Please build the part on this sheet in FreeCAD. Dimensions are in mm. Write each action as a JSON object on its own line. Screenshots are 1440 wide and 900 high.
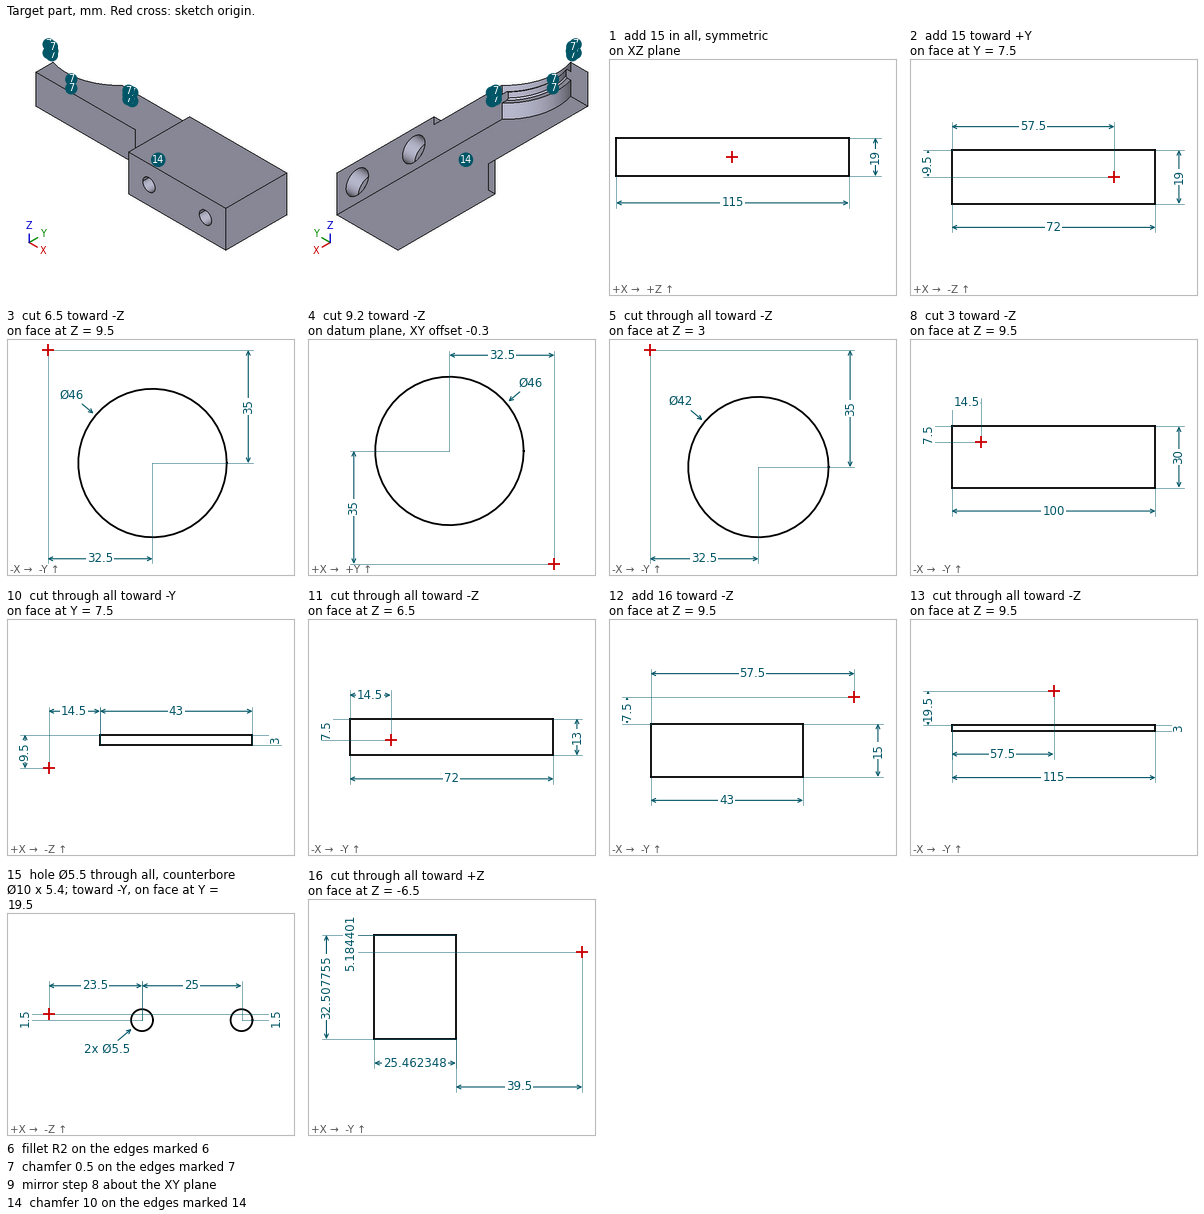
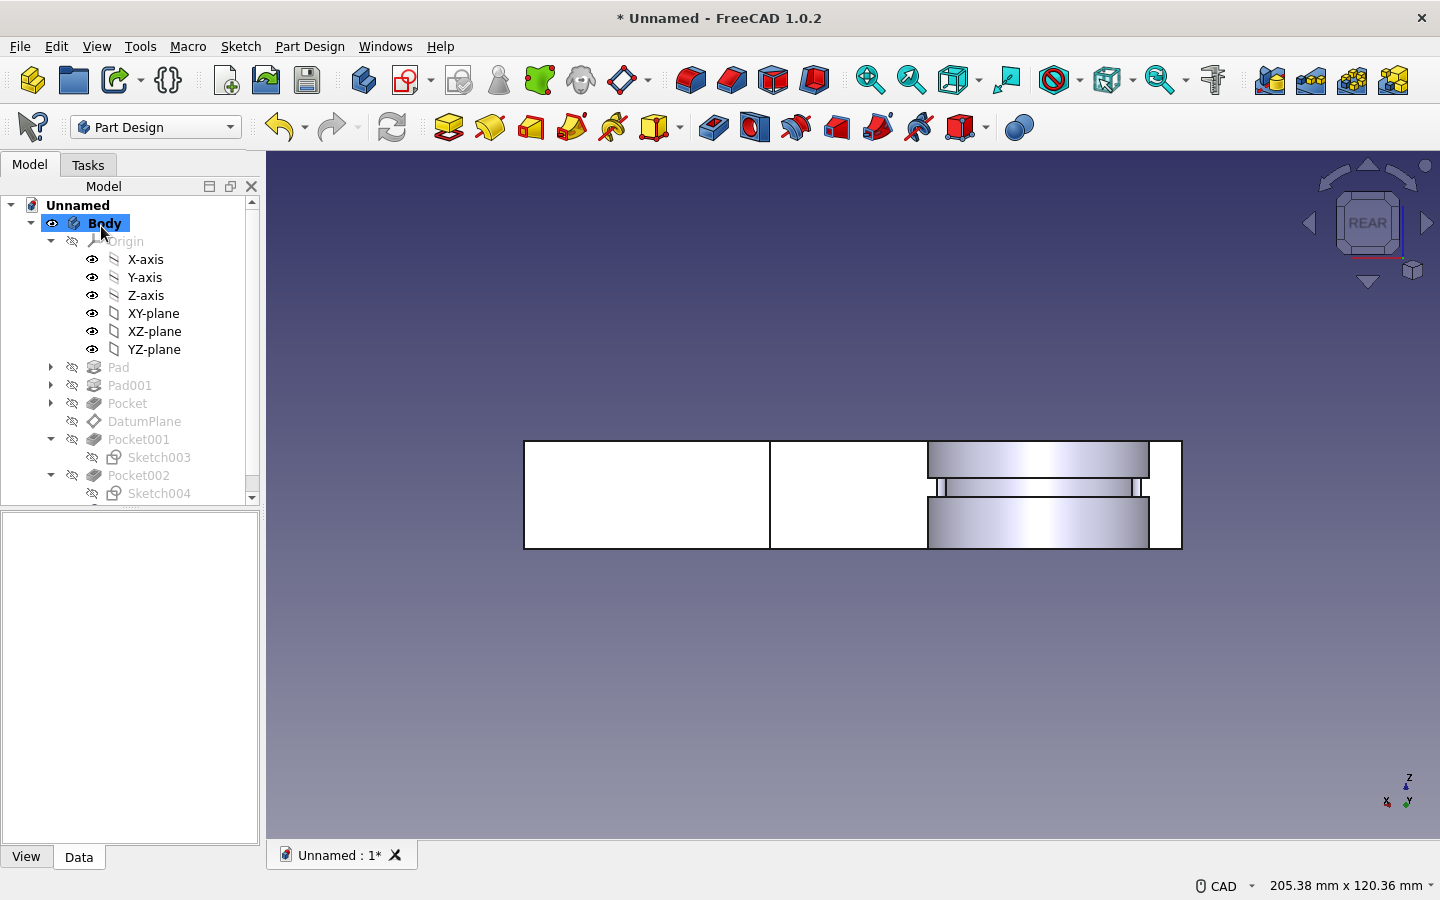
{"action": "left_click", "coordinate": [1060, 477]}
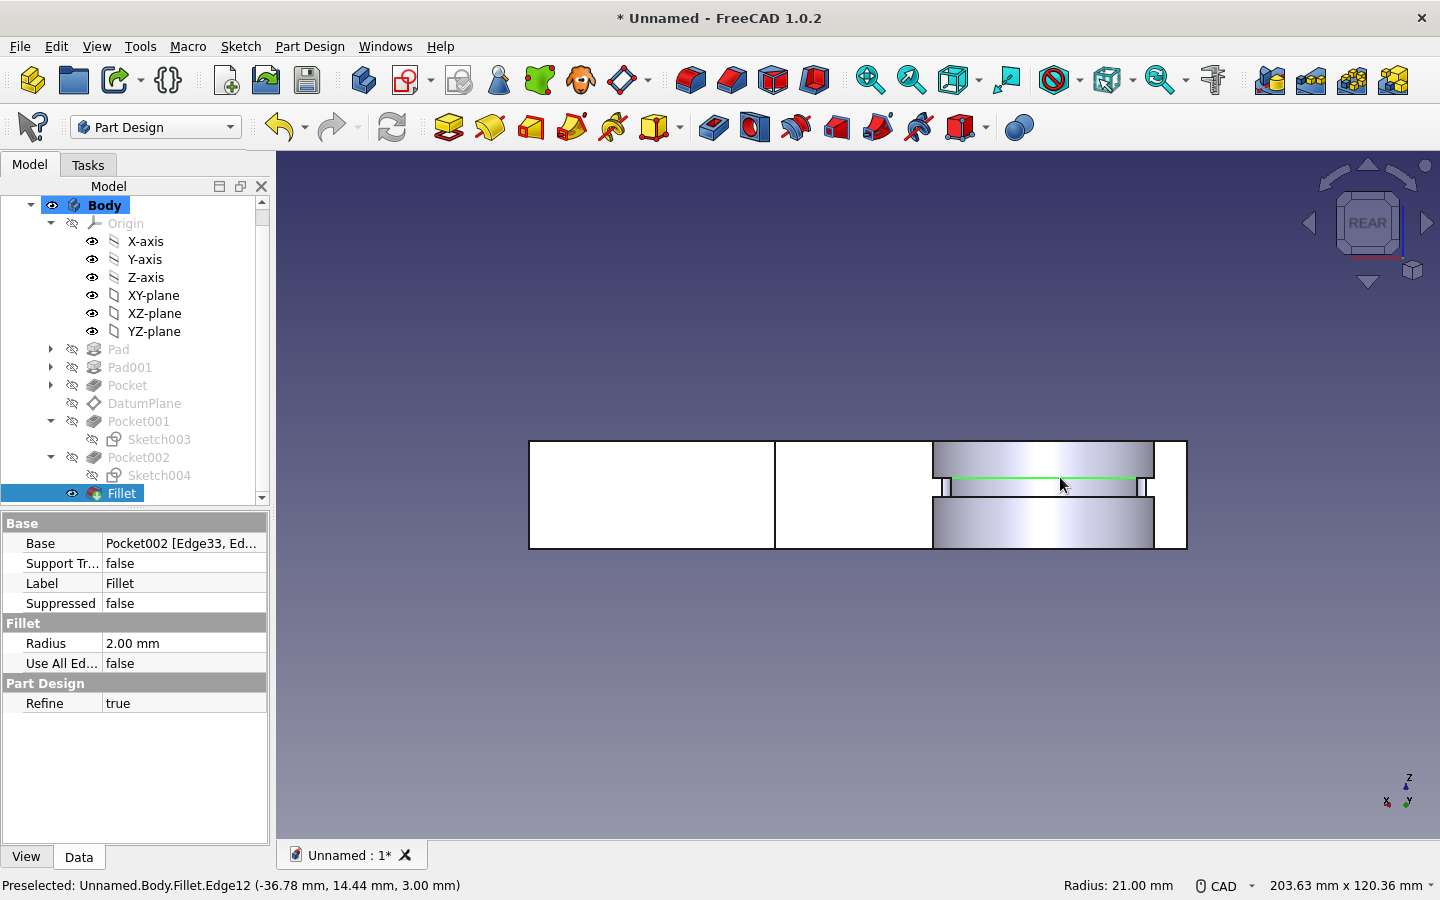
{"action": "left_click", "coordinate": [1044, 496], "text": "ctrl"}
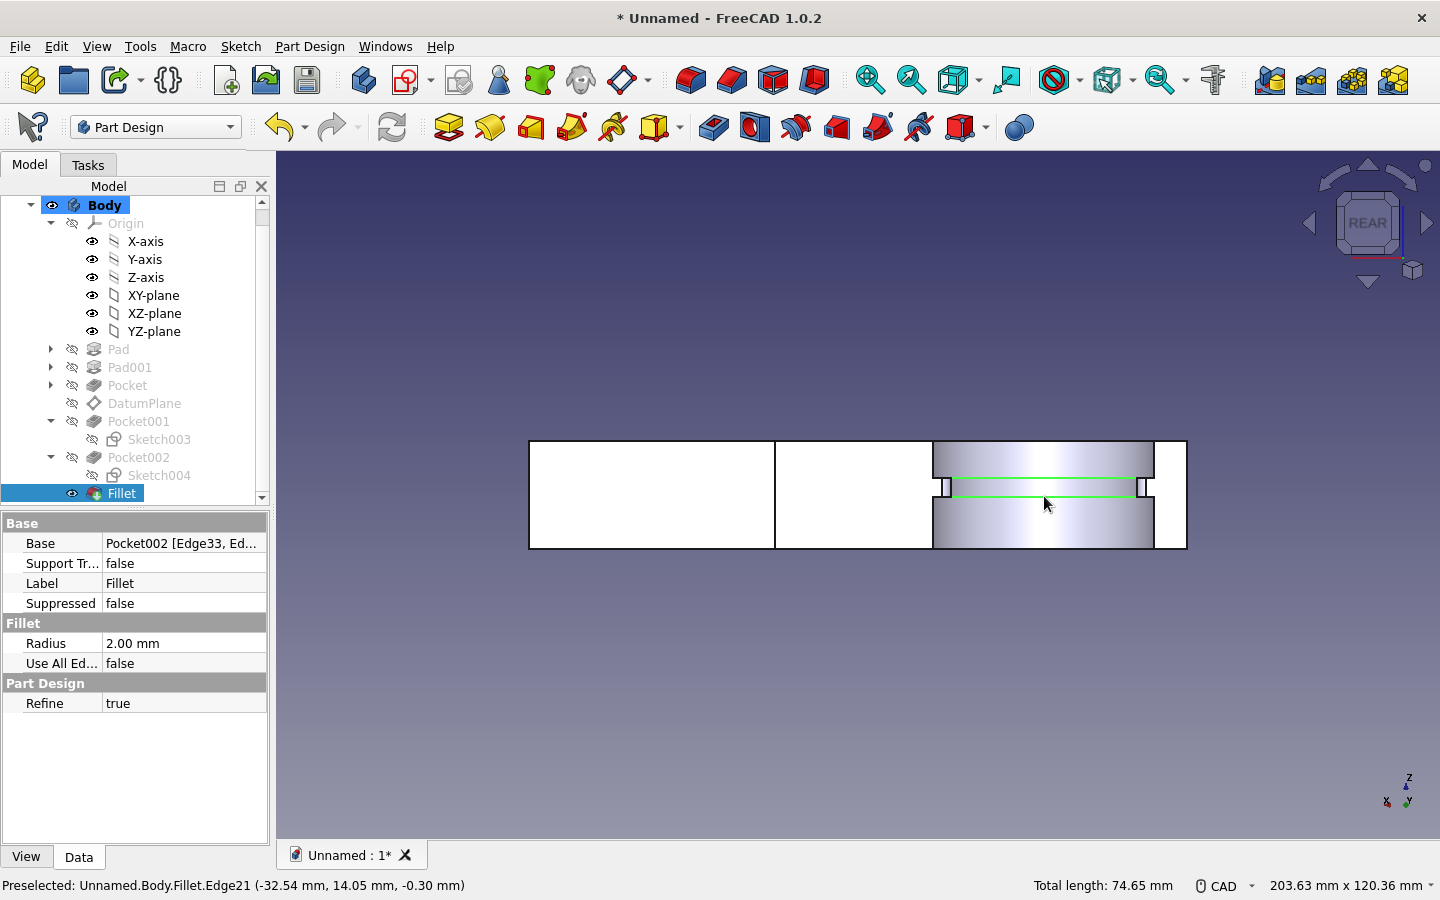
{"action": "left_click", "coordinate": [1139, 496], "text": "ctrl"}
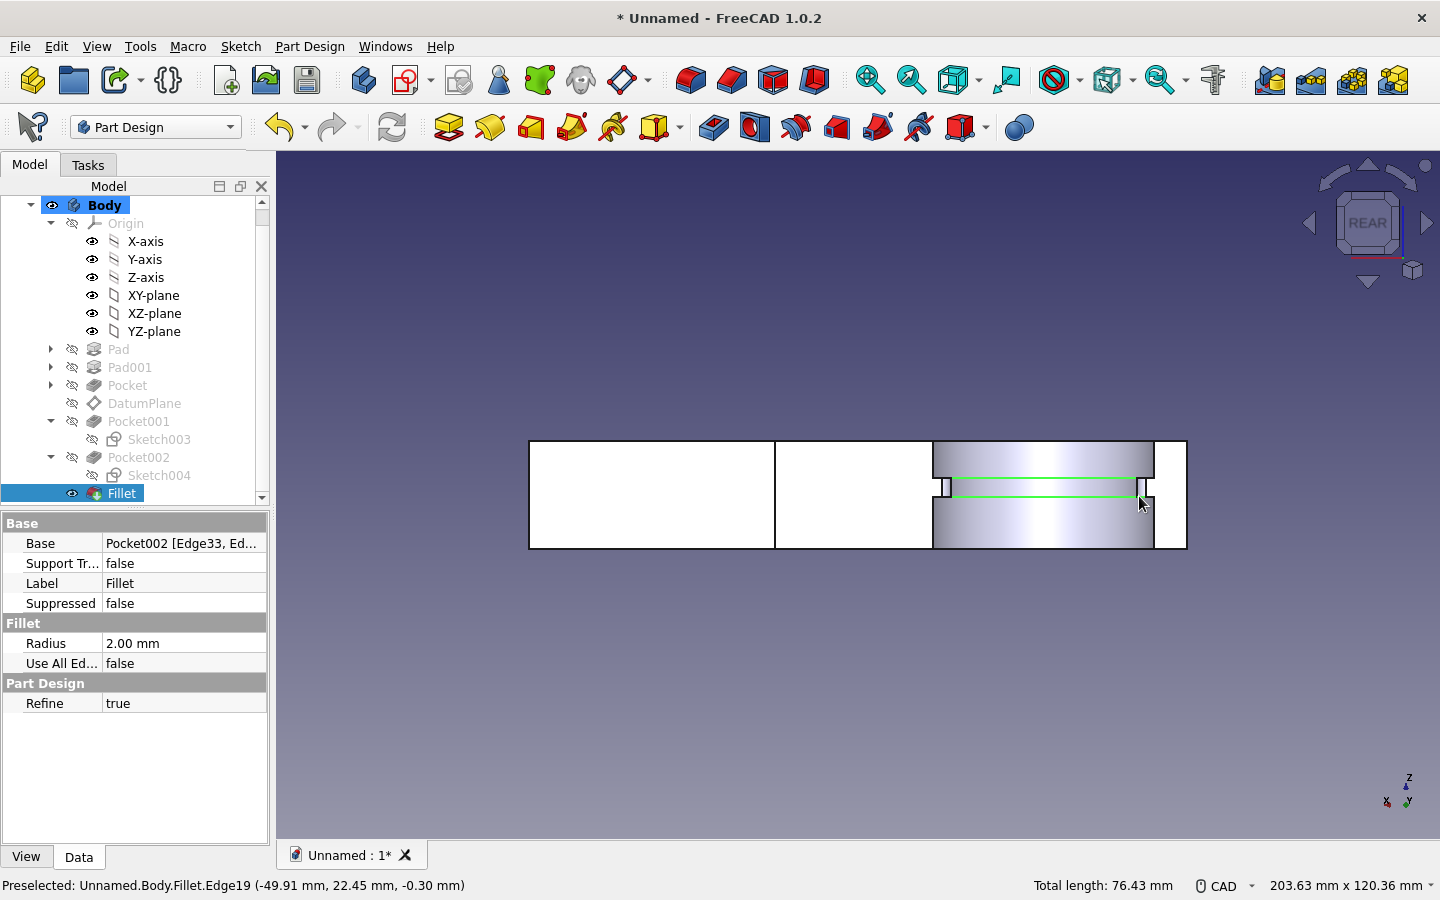
{"action": "left_click", "coordinate": [948, 496], "text": "ctrl"}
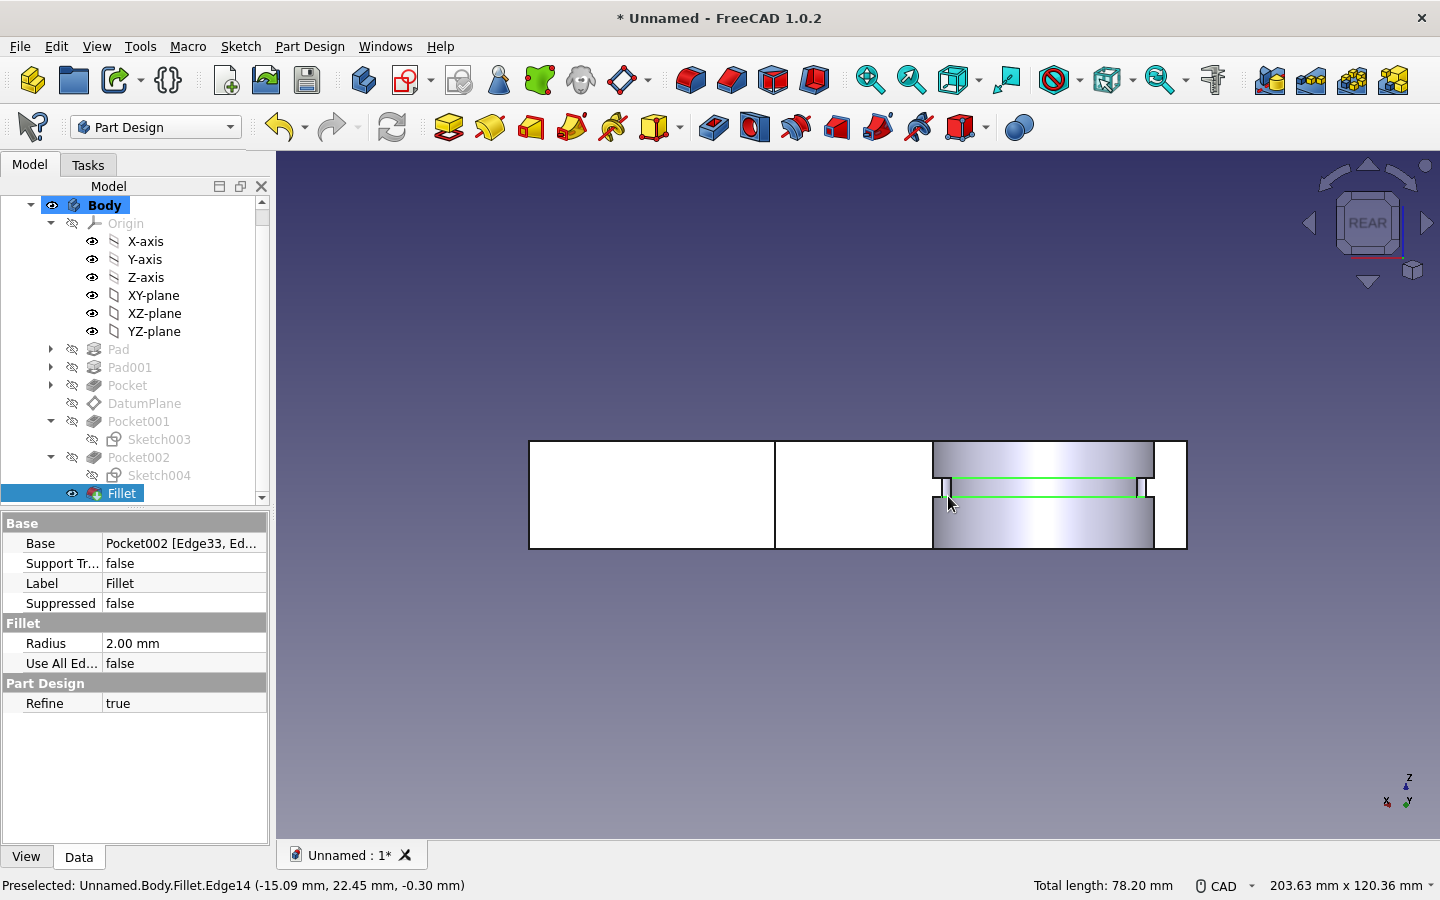
{"action": "left_click", "coordinate": [1139, 477], "text": "ctrl"}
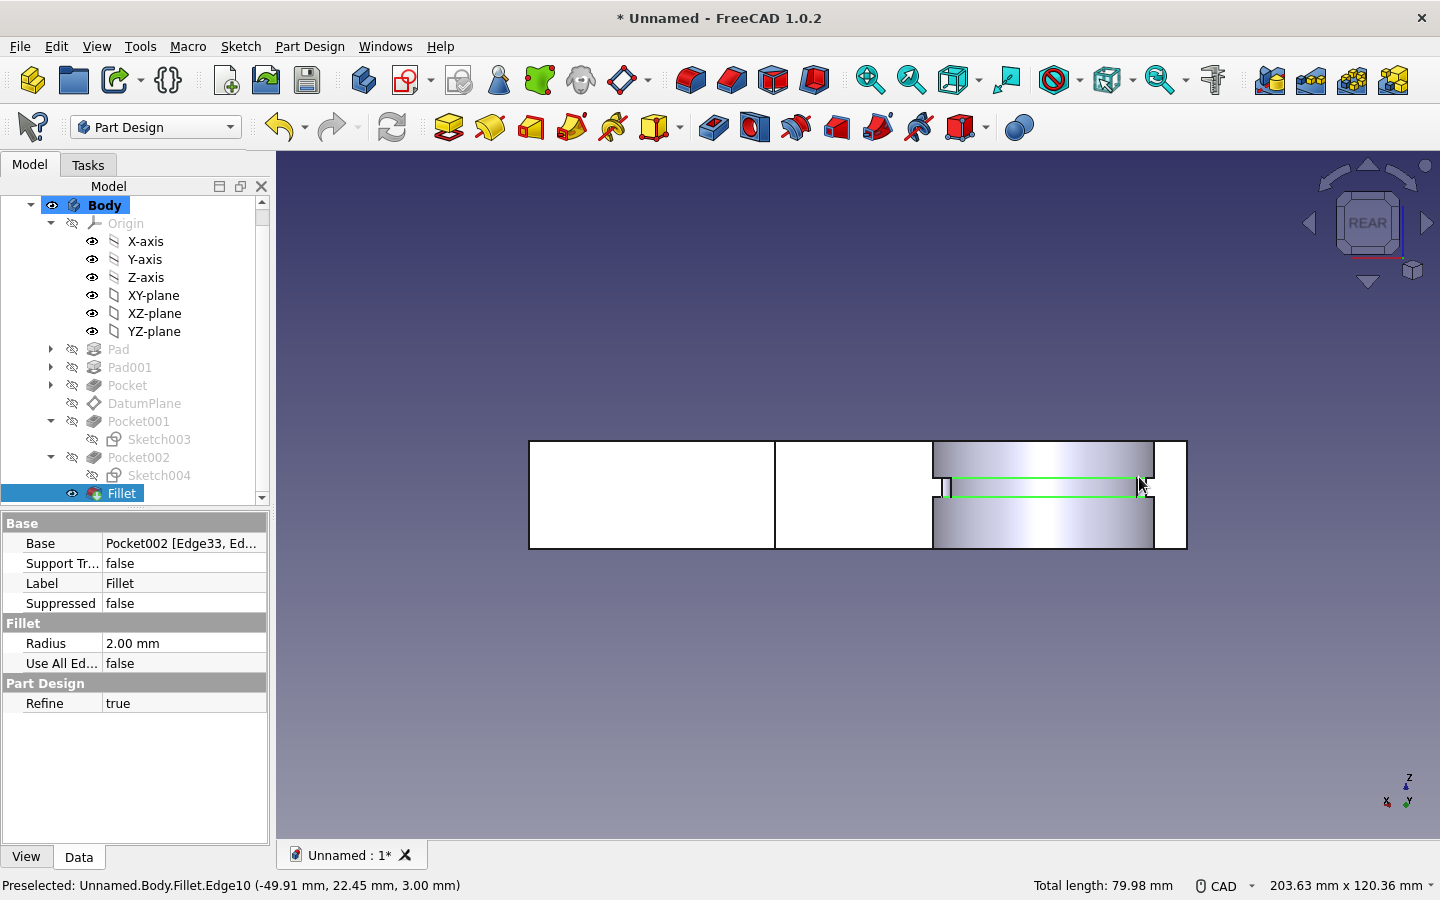
{"action": "left_click", "coordinate": [948, 477], "text": "ctrl"}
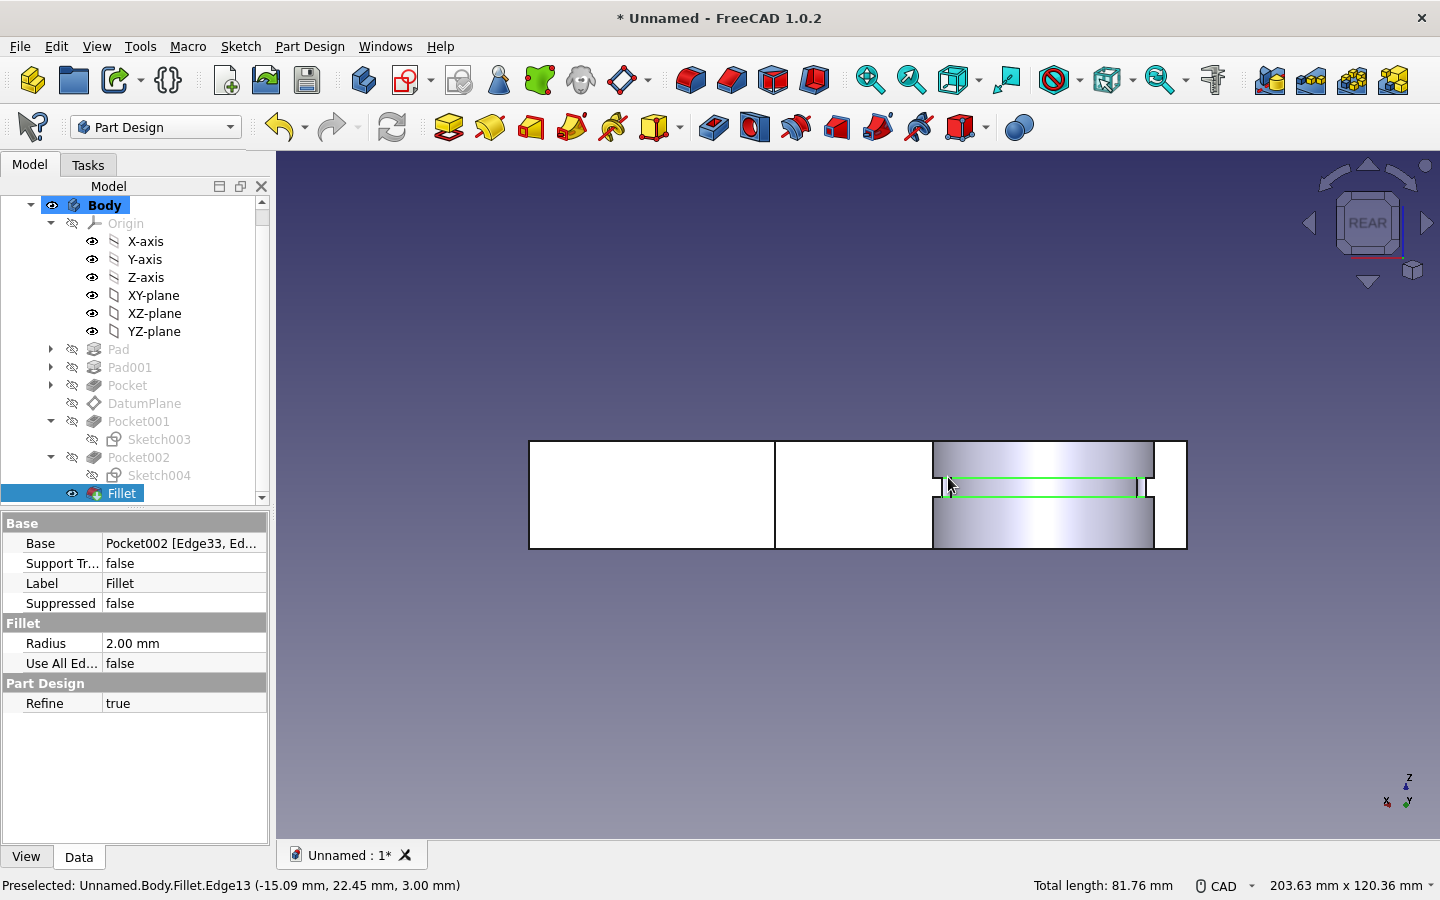
{"action": "scroll", "coordinate": [1150, 477], "scroll_direction": "up", "scroll_amount": 8}